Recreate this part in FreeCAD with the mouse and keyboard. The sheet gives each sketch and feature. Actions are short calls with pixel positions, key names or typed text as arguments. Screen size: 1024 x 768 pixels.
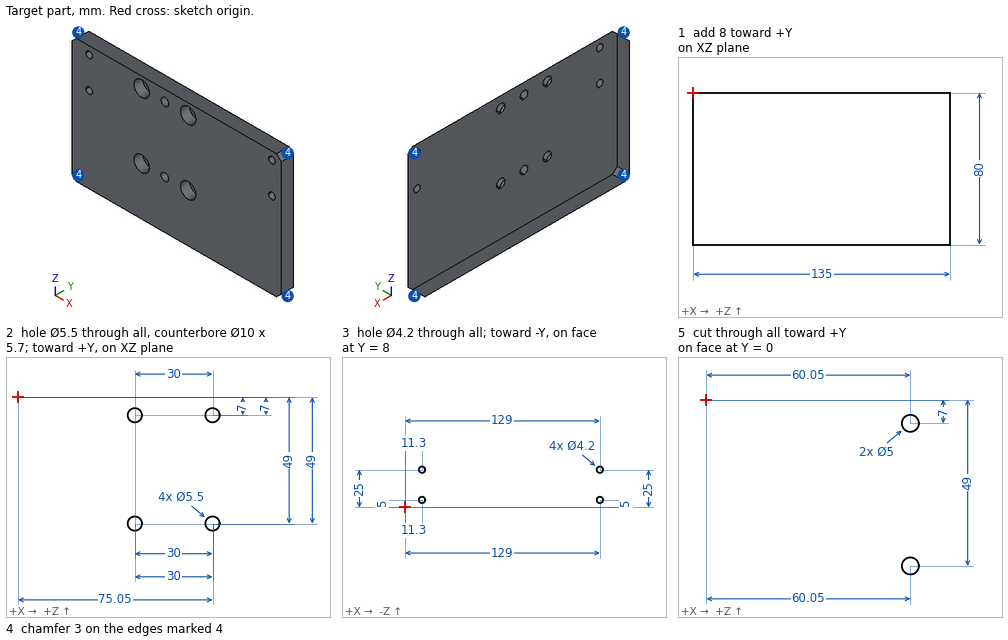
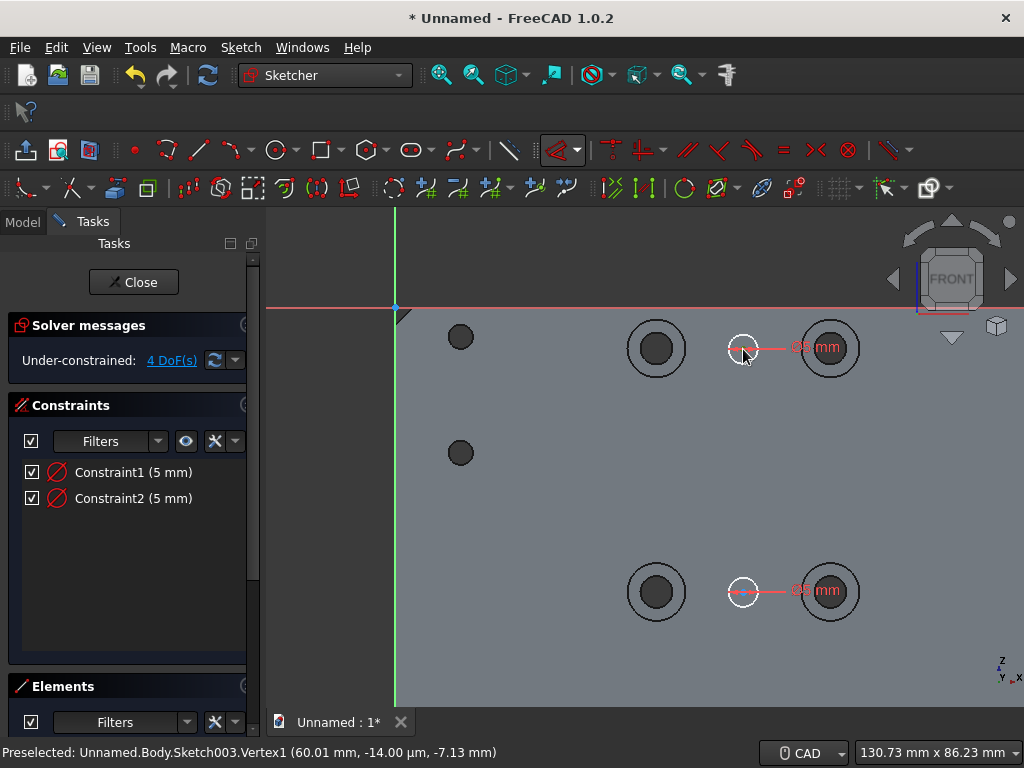
key(i)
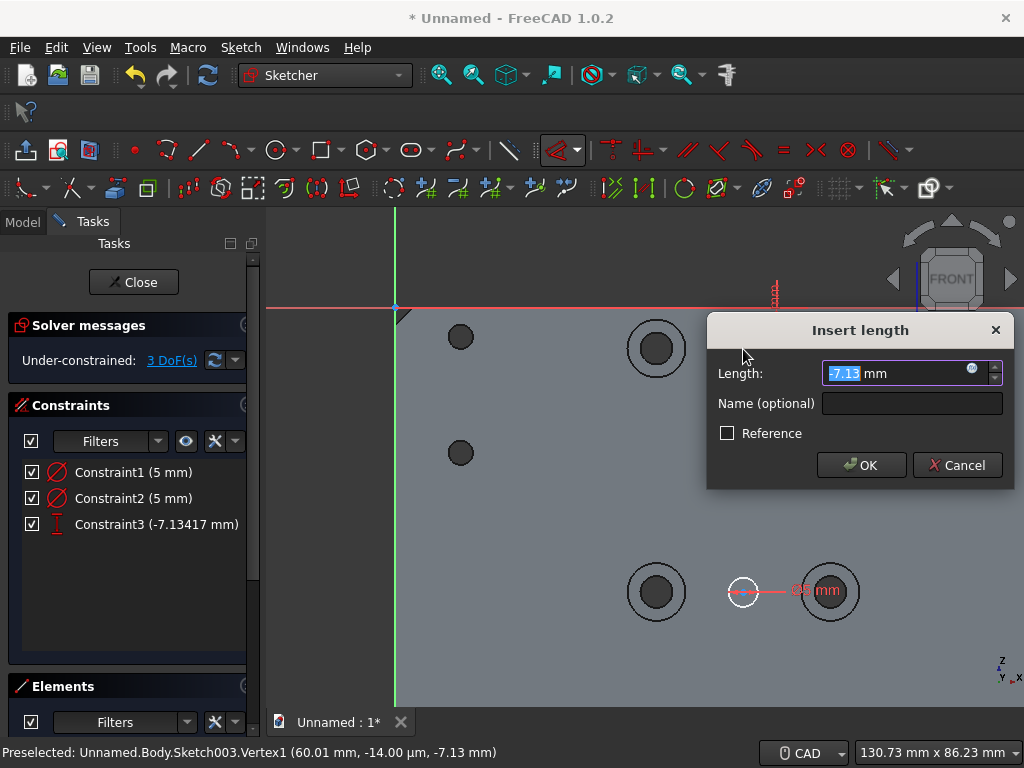
text(-7)
key(Return)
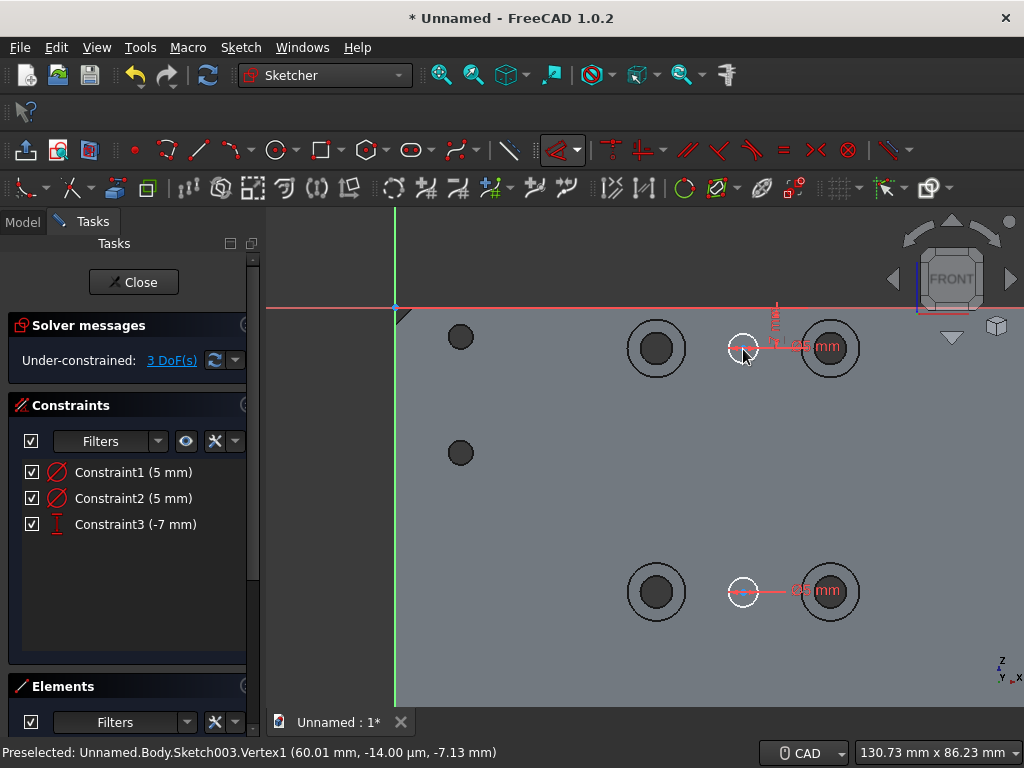
click(743, 592)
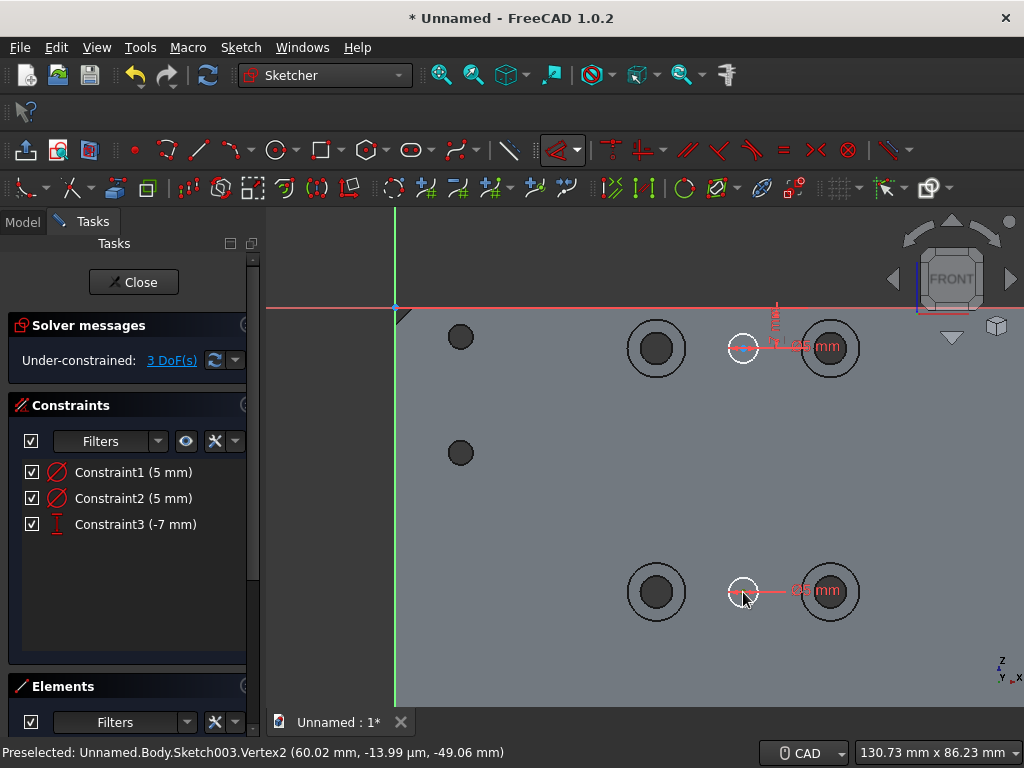
key(i)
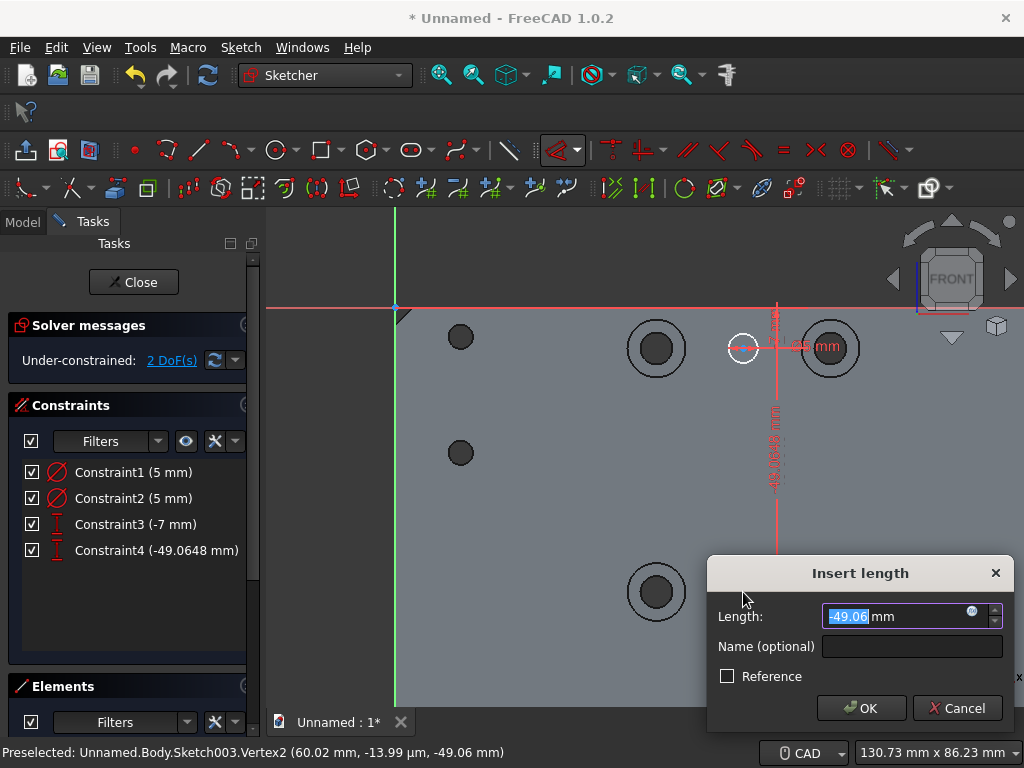
text(-49)
key(Return)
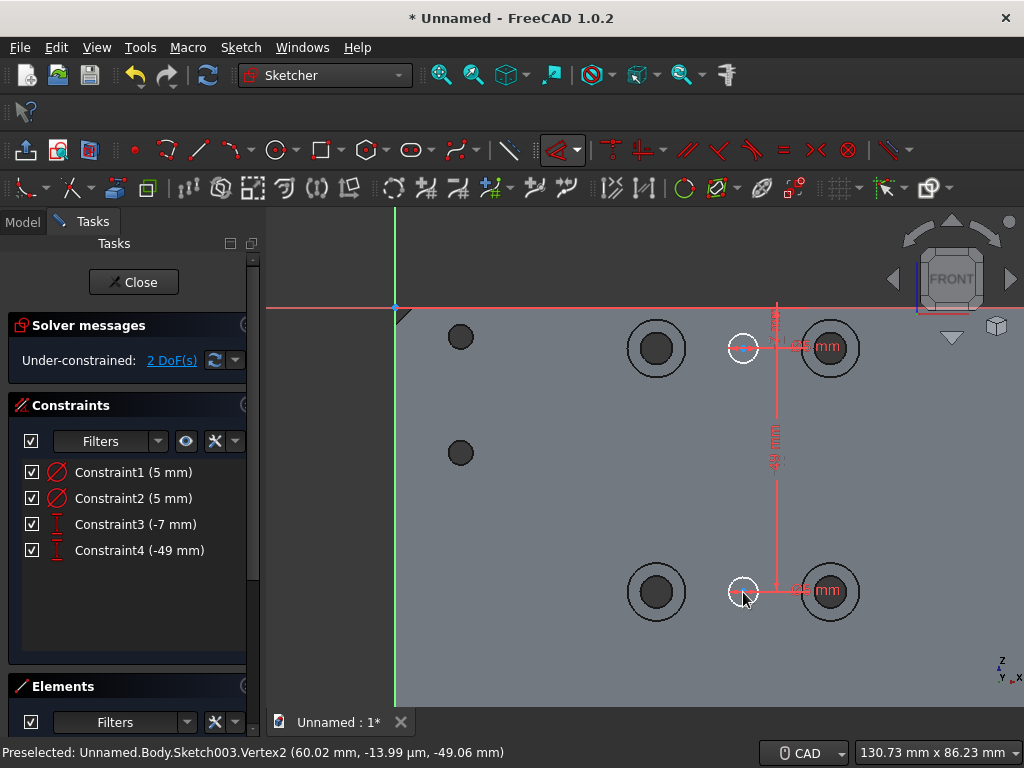
click(743, 348)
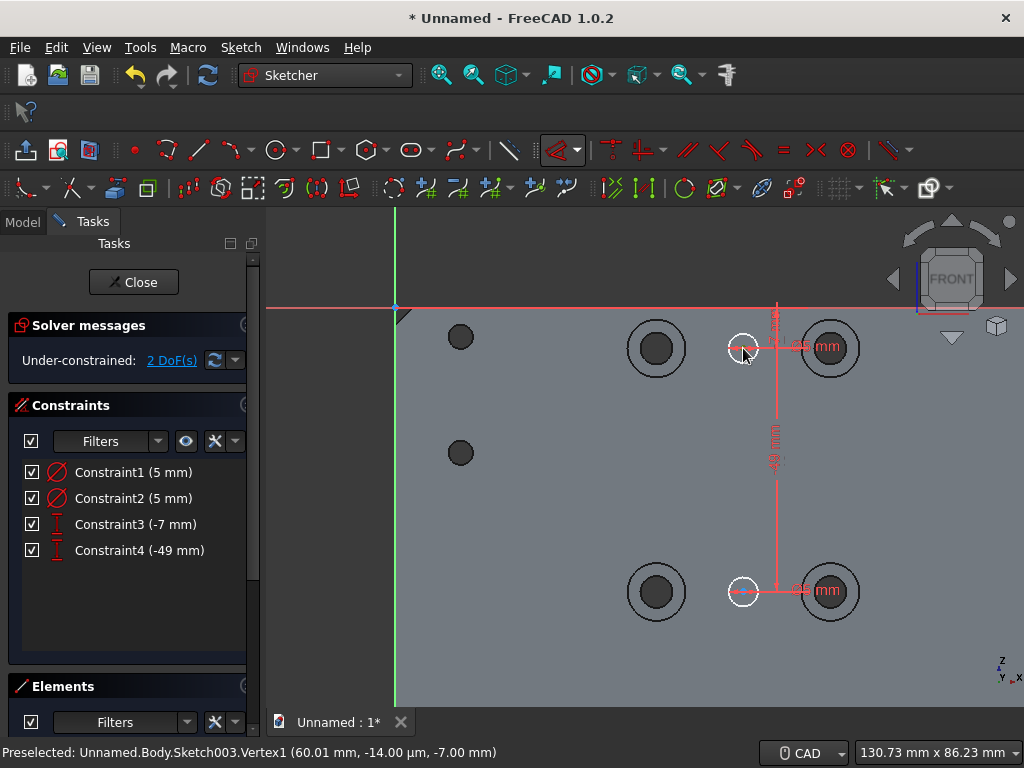
key(l)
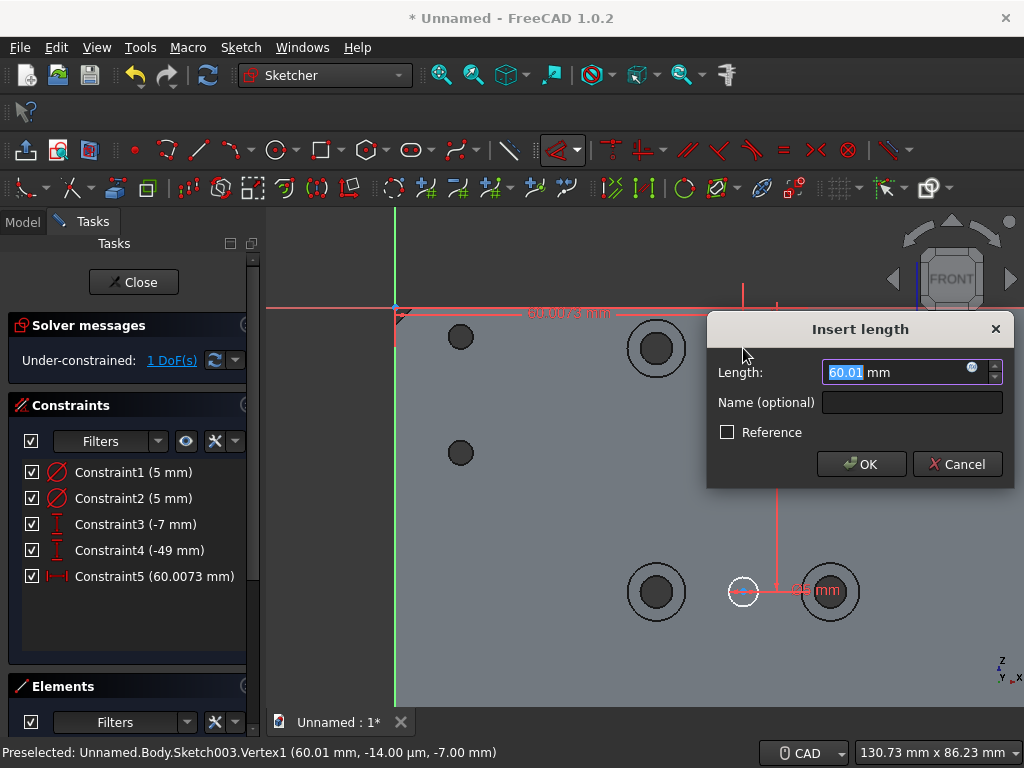
text(60.05)
key(Return)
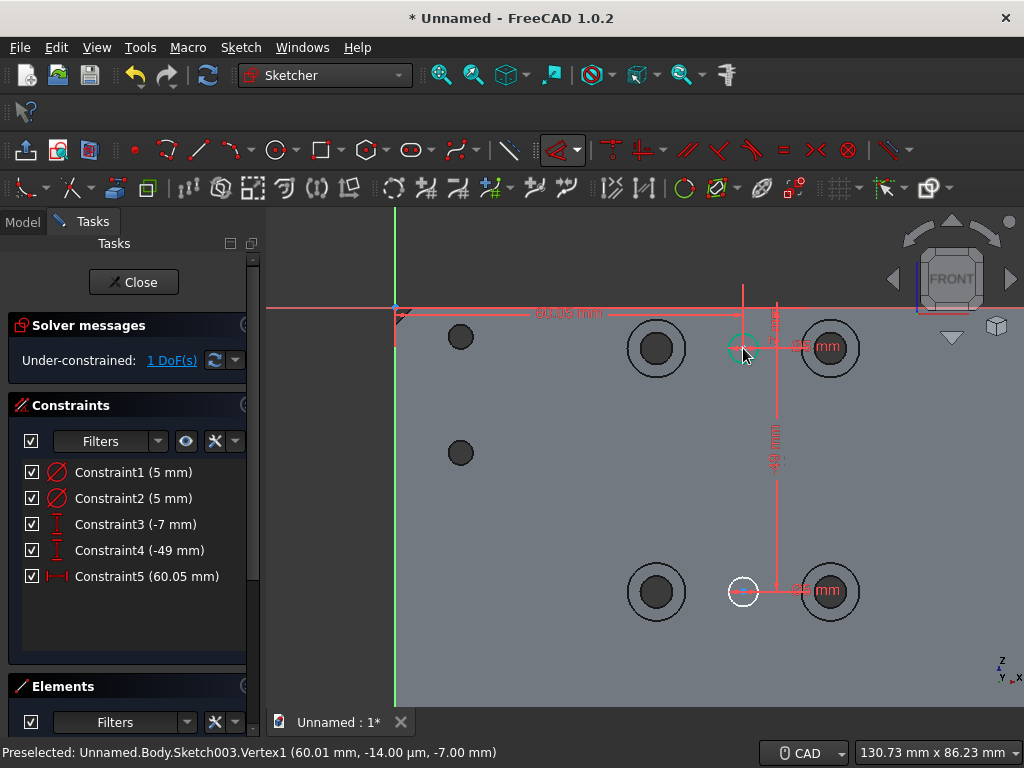
click(743, 592)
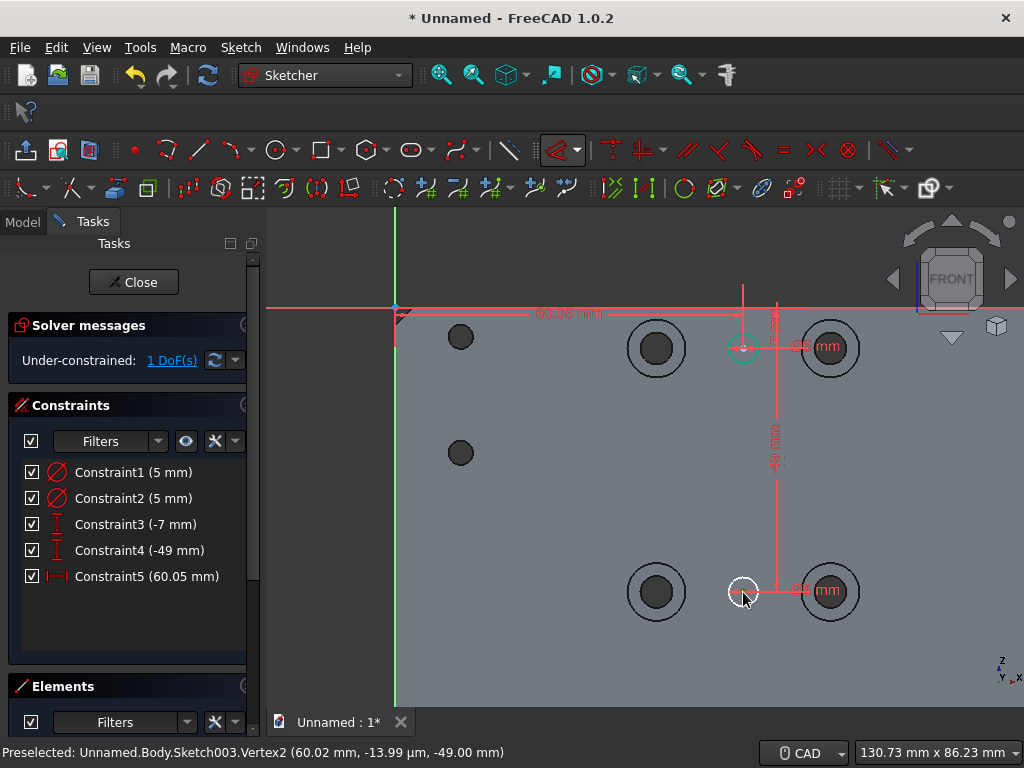
key(l)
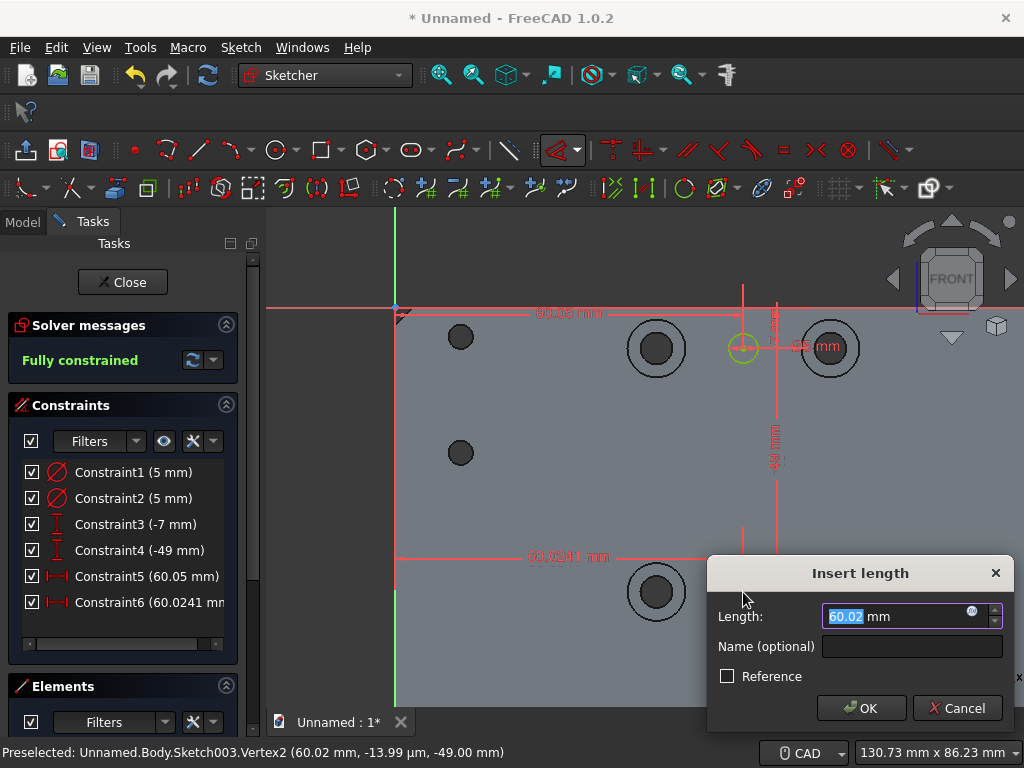
text(60.05)
key(Return)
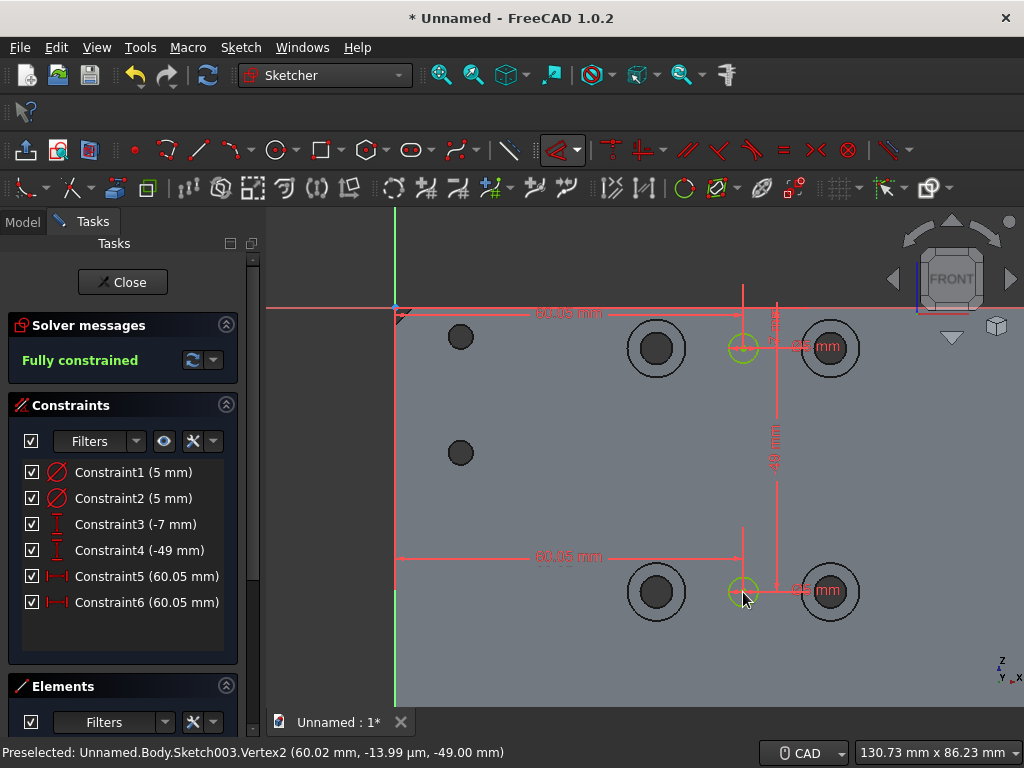
click(123, 282)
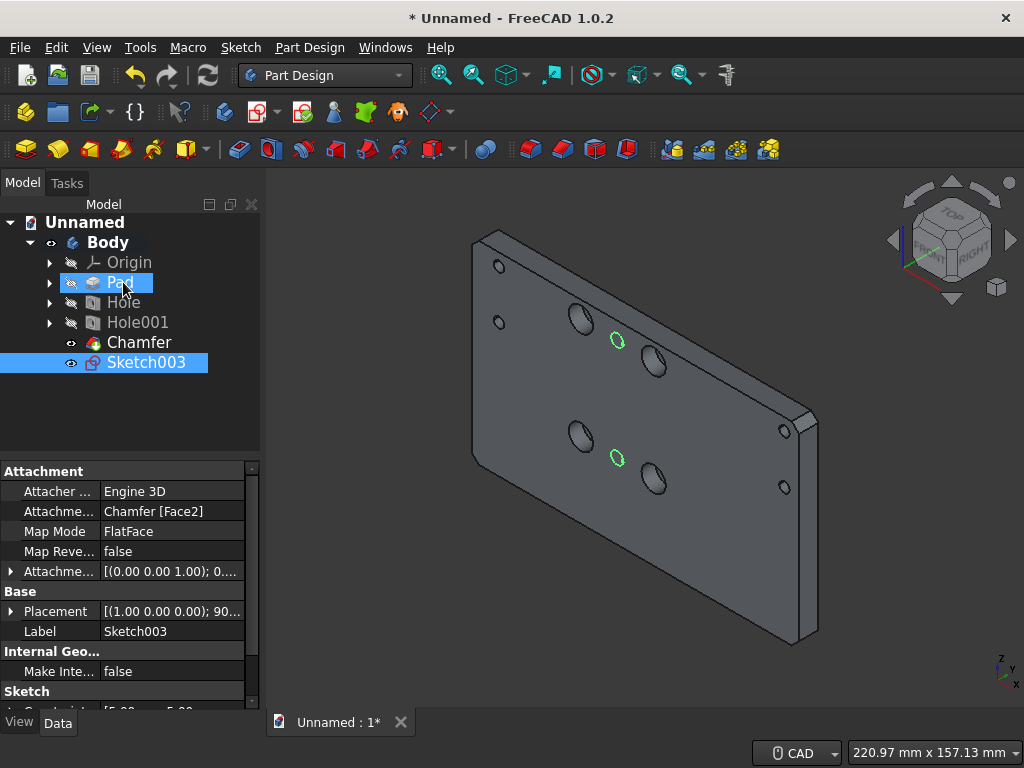
click(240, 150)